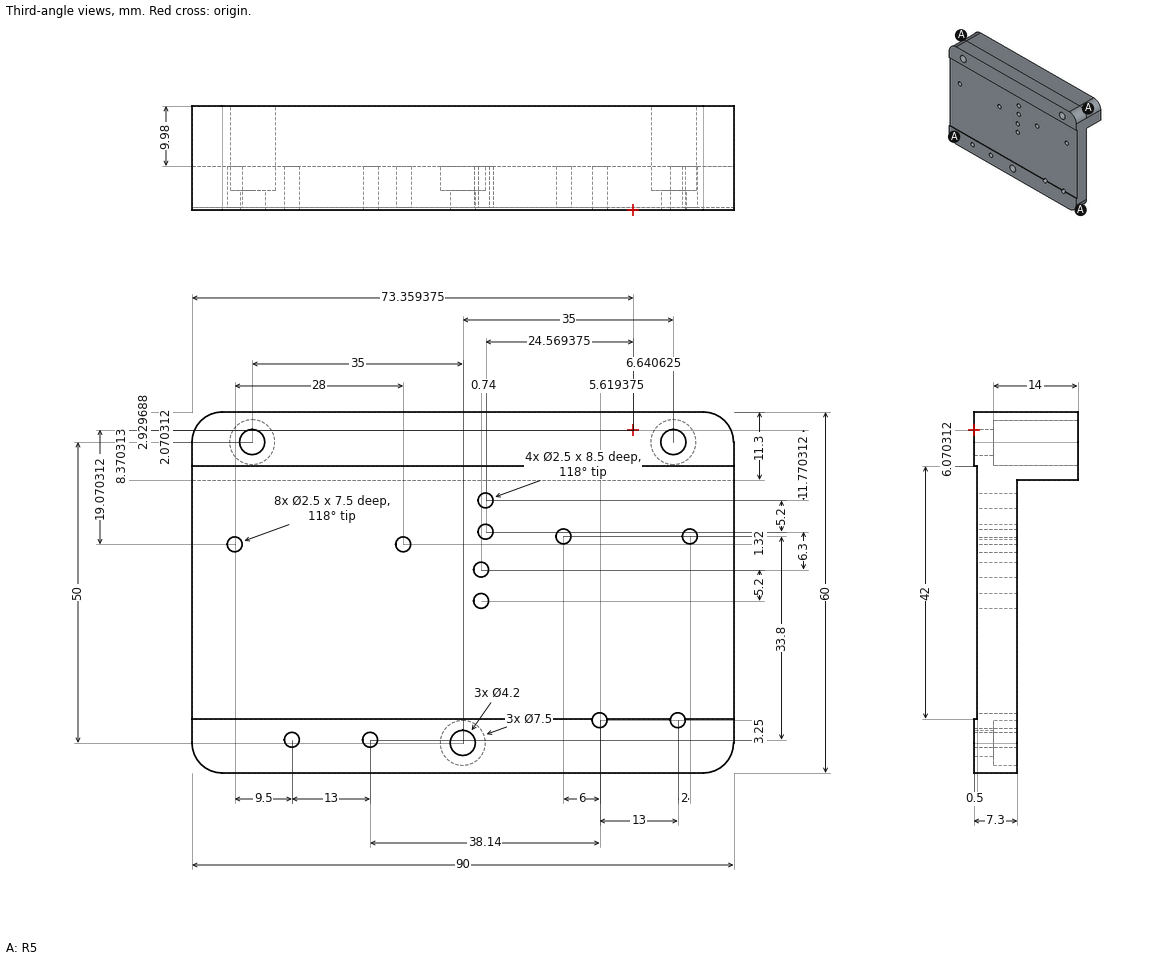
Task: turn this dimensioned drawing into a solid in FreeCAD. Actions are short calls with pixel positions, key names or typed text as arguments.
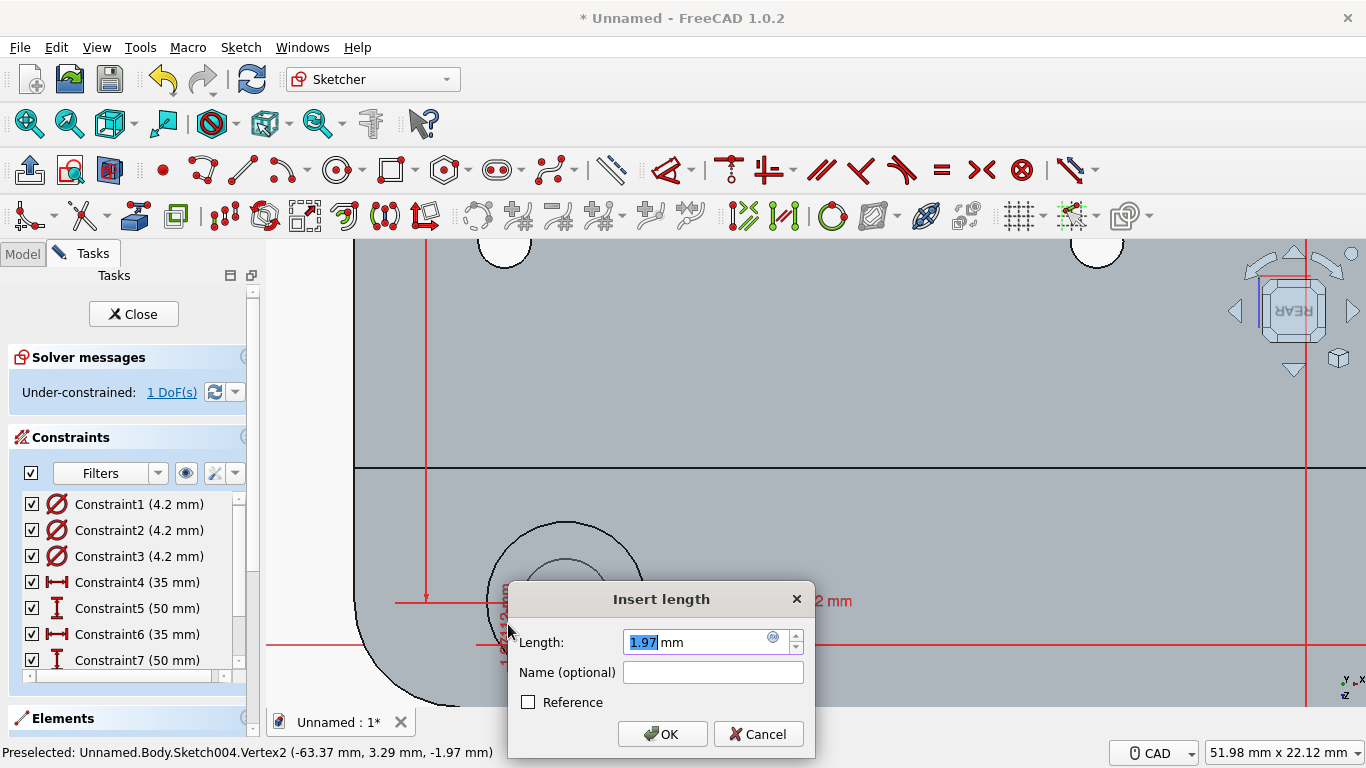
text(2.070312)
key(Return)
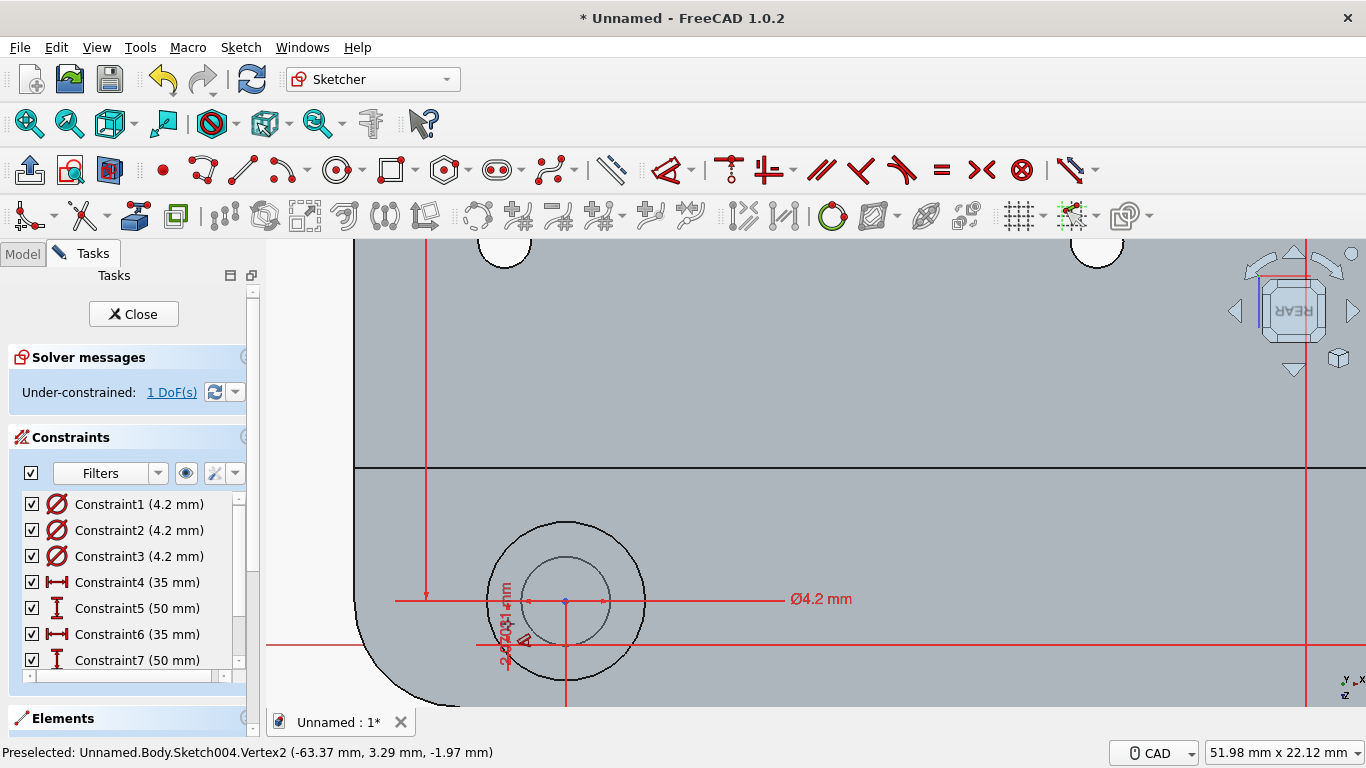
scroll(564, 604, down, 7)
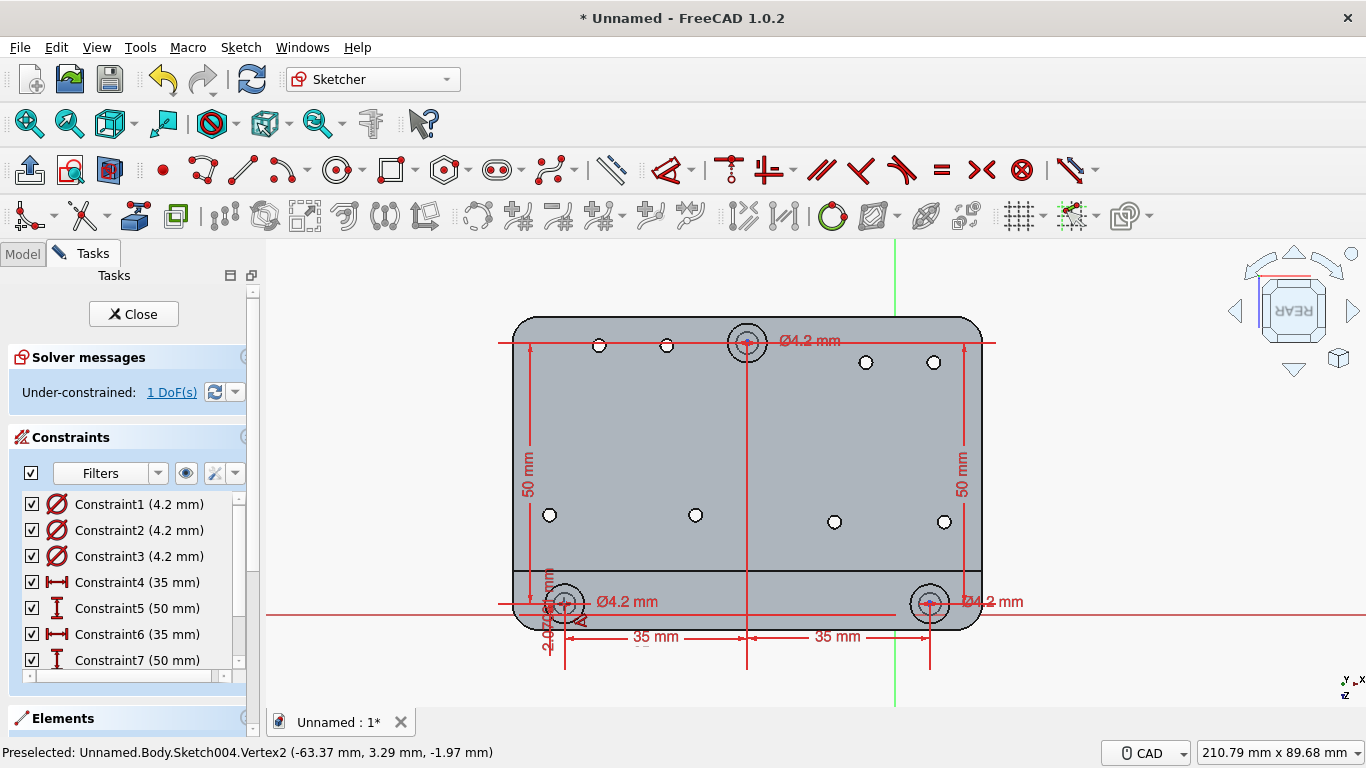
click(930, 604)
click(913, 649)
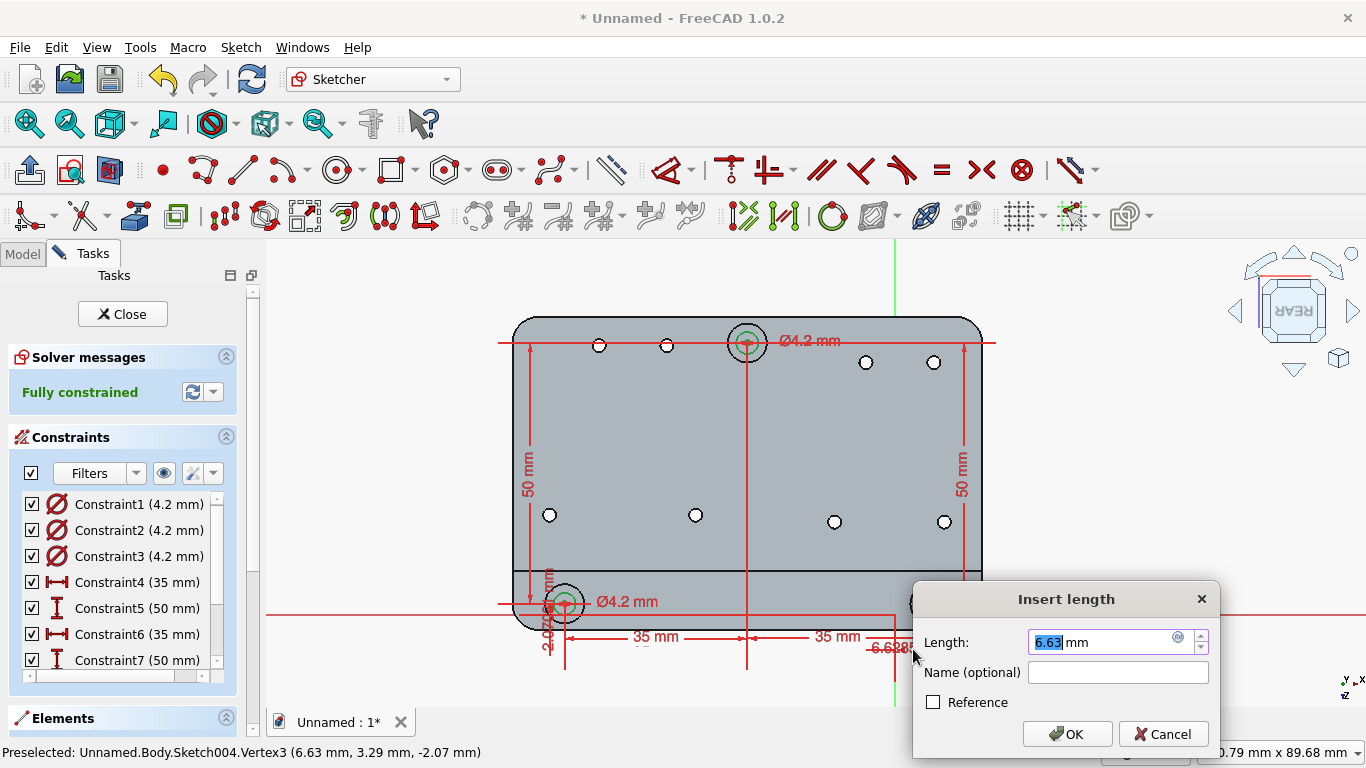
text(6.640625)
key(Return)
key(Escape)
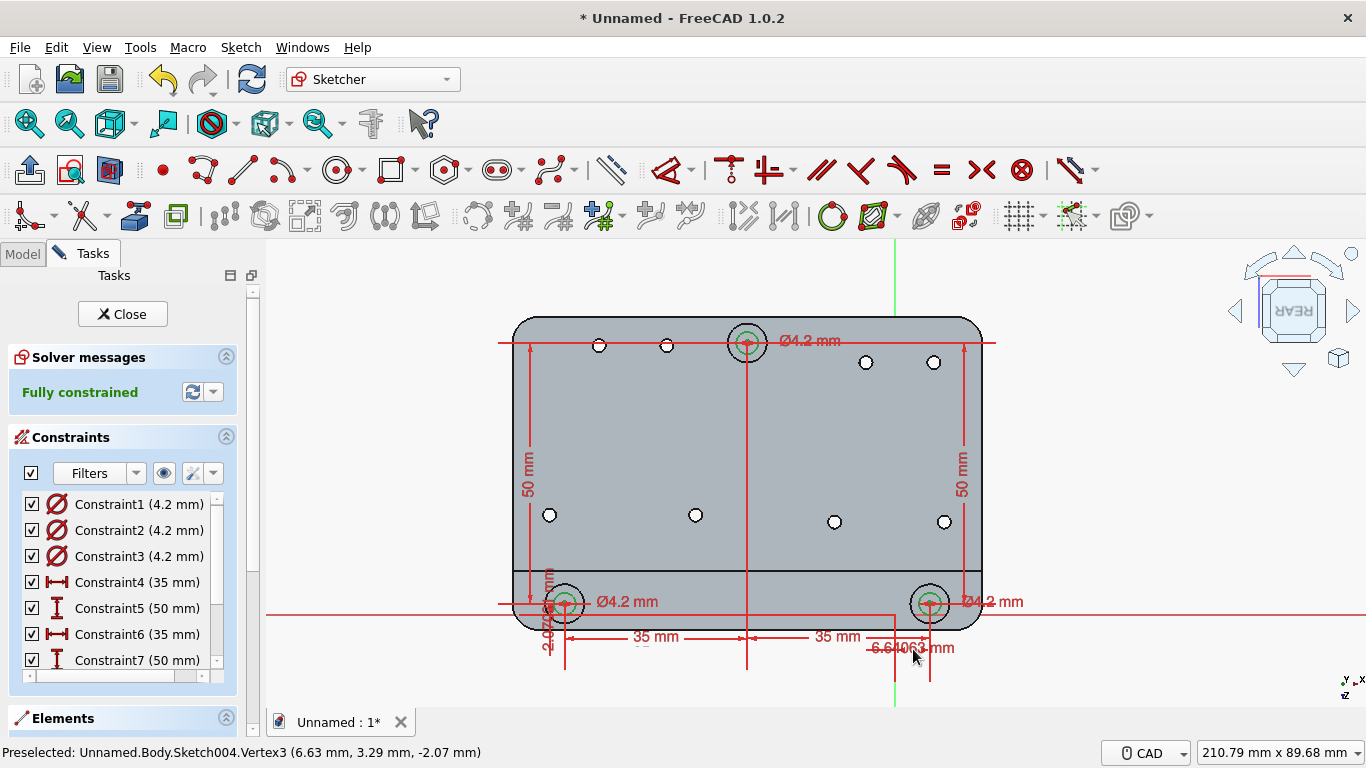
click(123, 314)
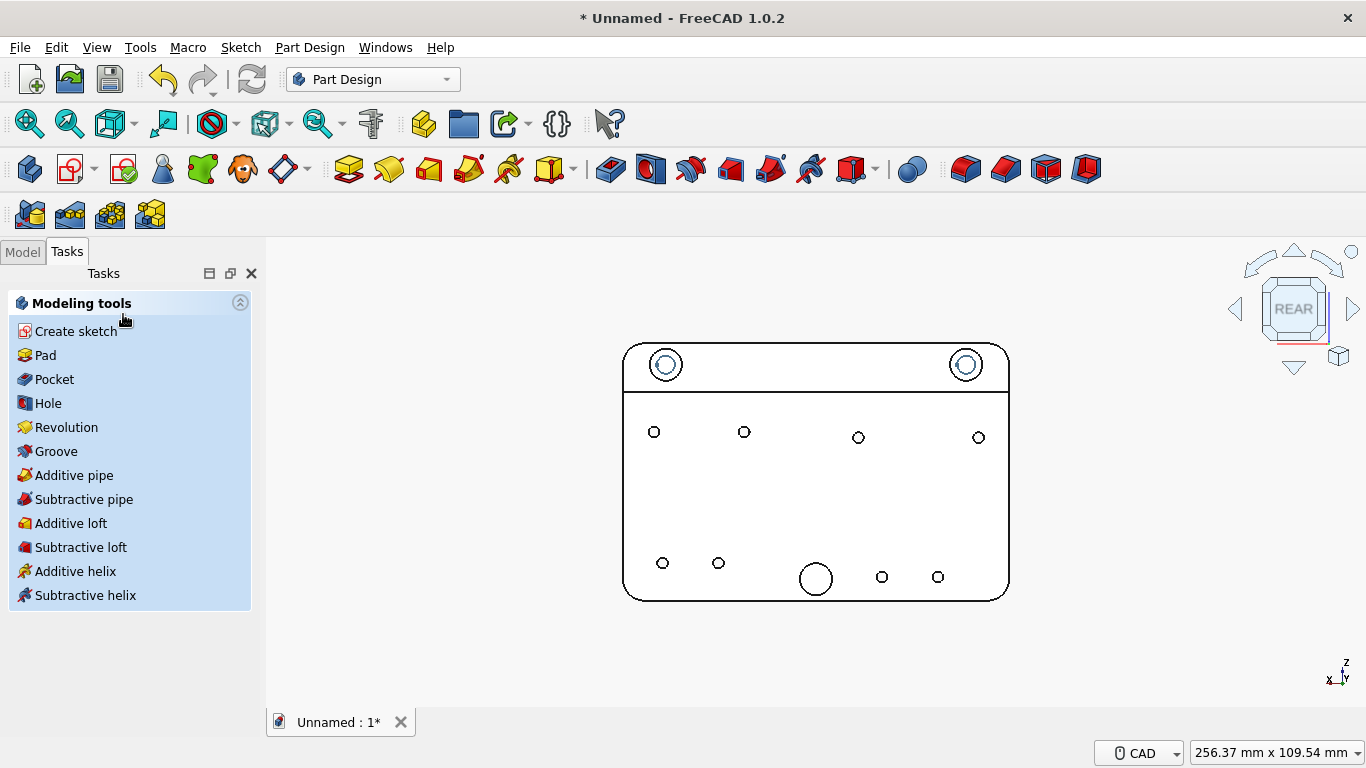
click(612, 170)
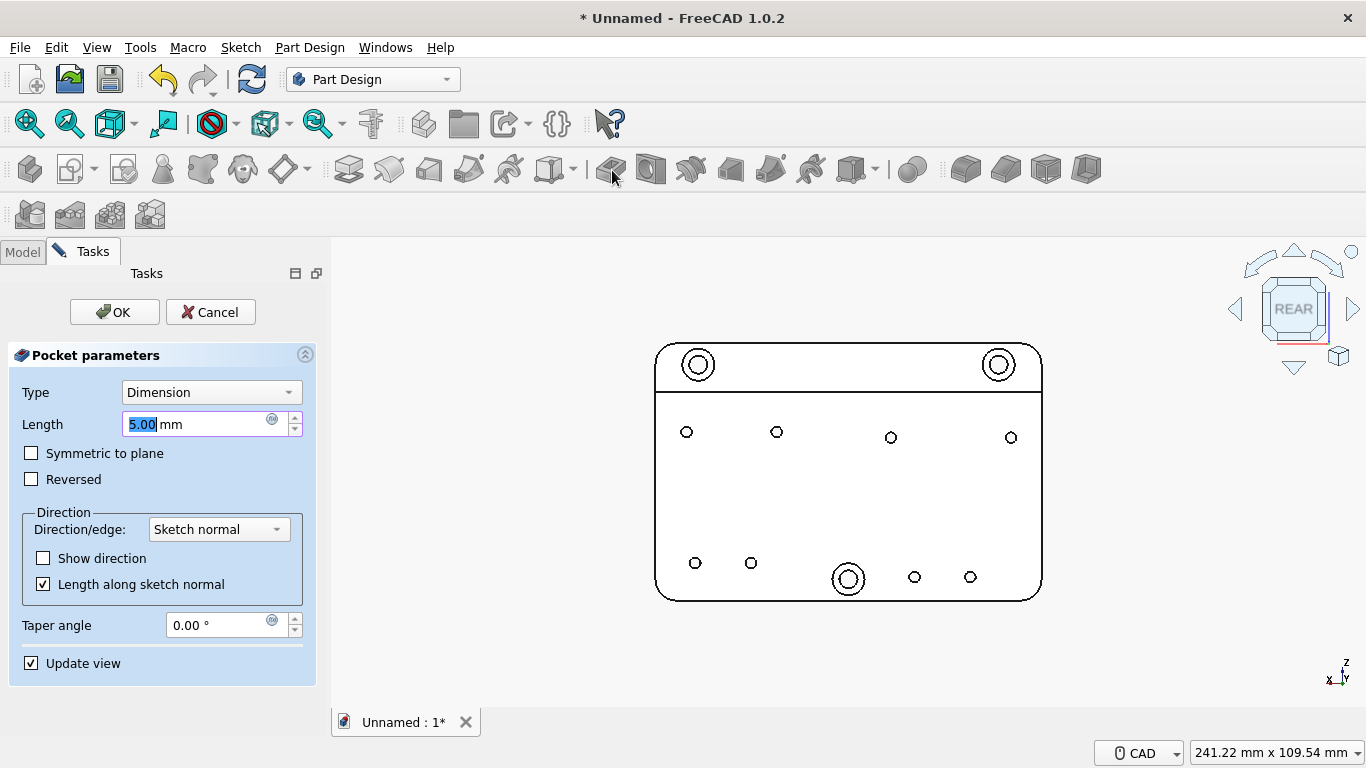
click(212, 392)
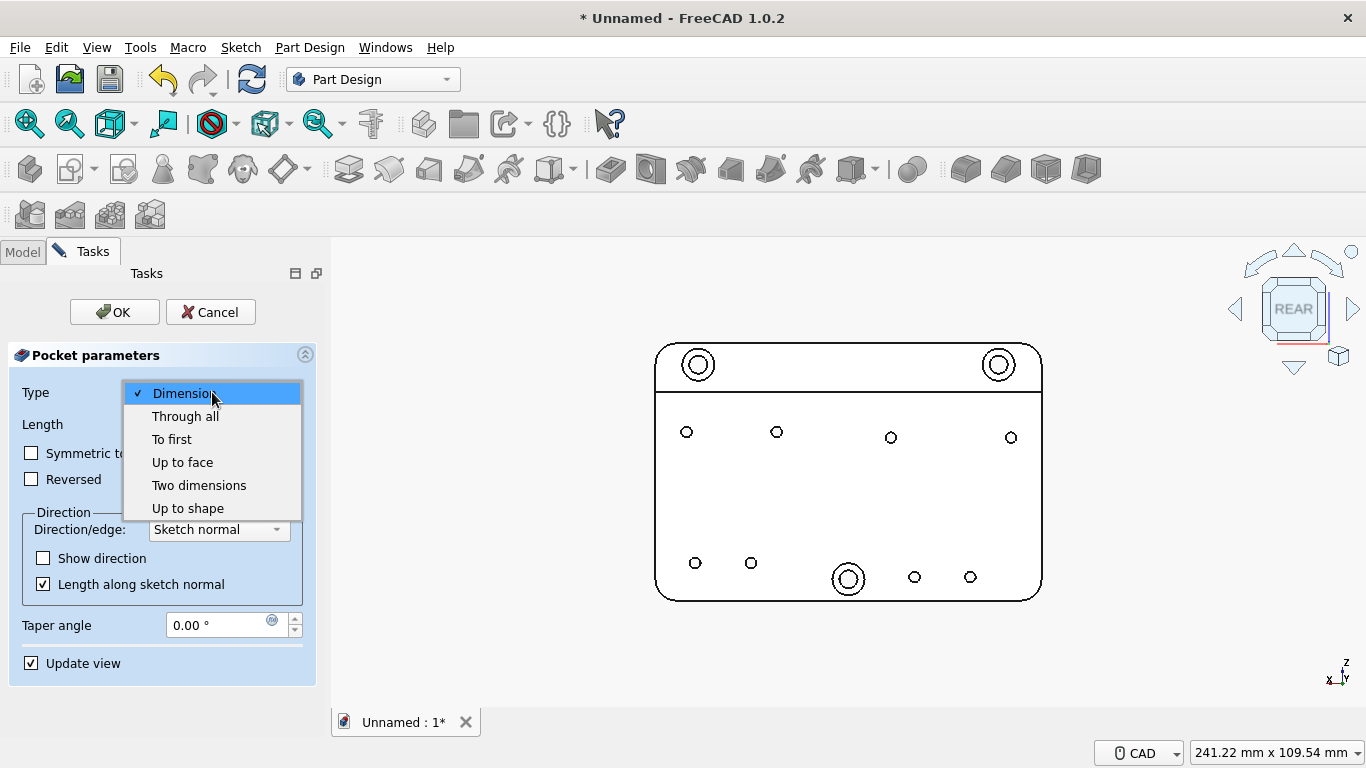
click(212, 416)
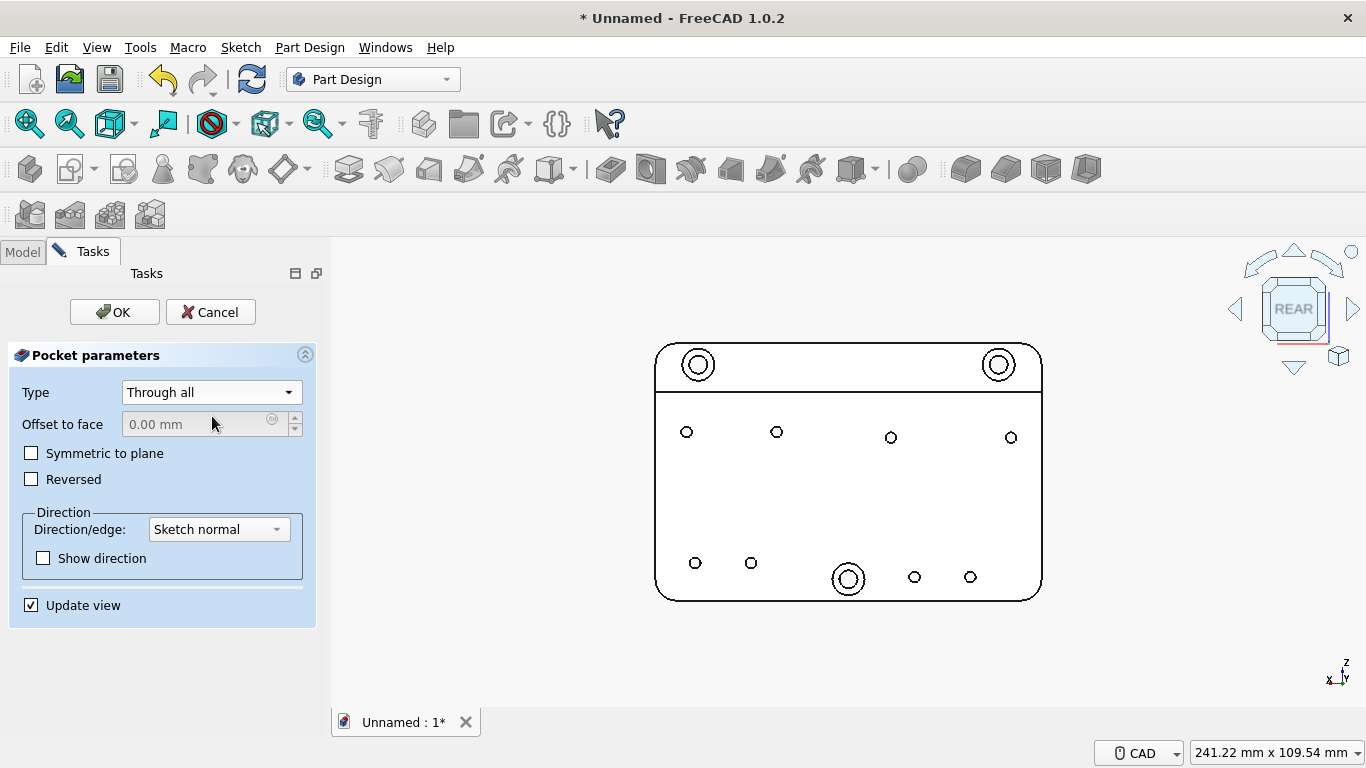
click(115, 312)